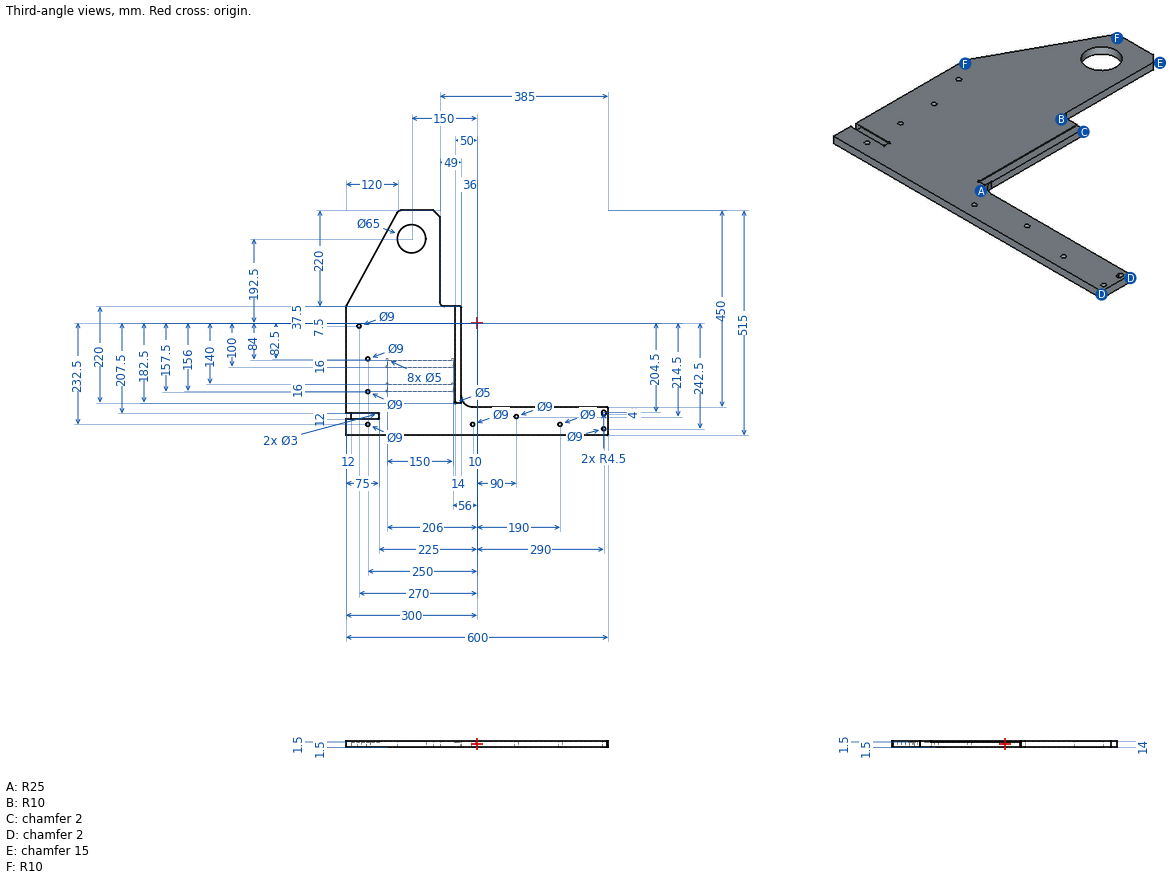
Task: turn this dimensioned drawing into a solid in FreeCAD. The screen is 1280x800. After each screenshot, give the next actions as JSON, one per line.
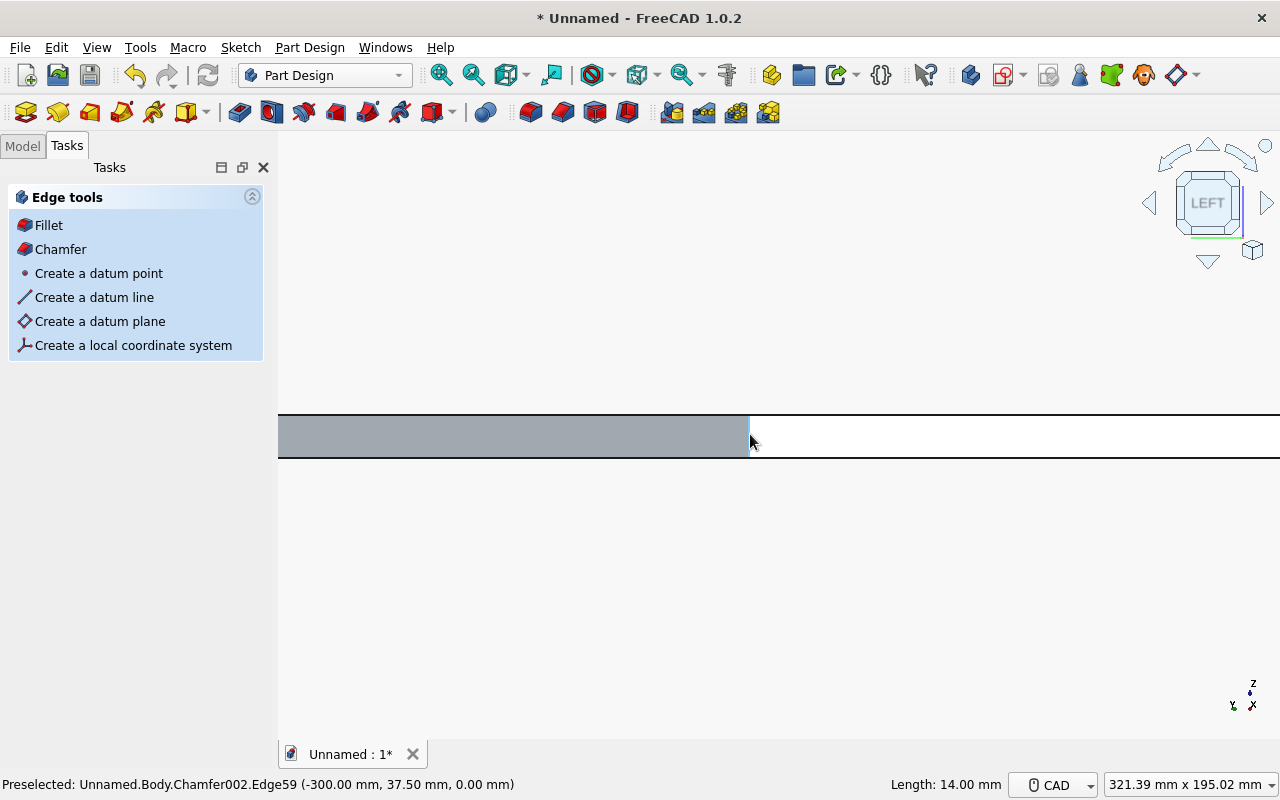
{"action": "left_click", "coordinate": [749, 436], "text": "ctrl"}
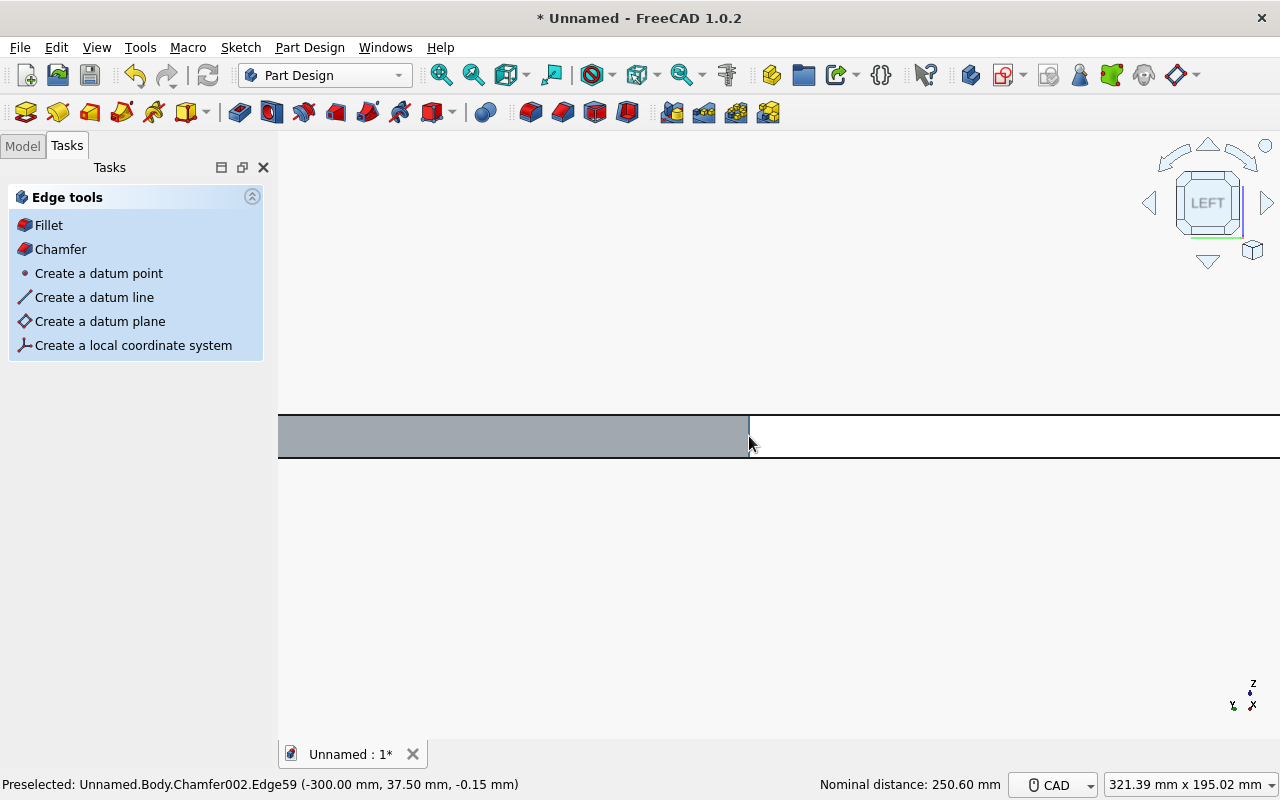
{"action": "left_click", "coordinate": [532, 112]}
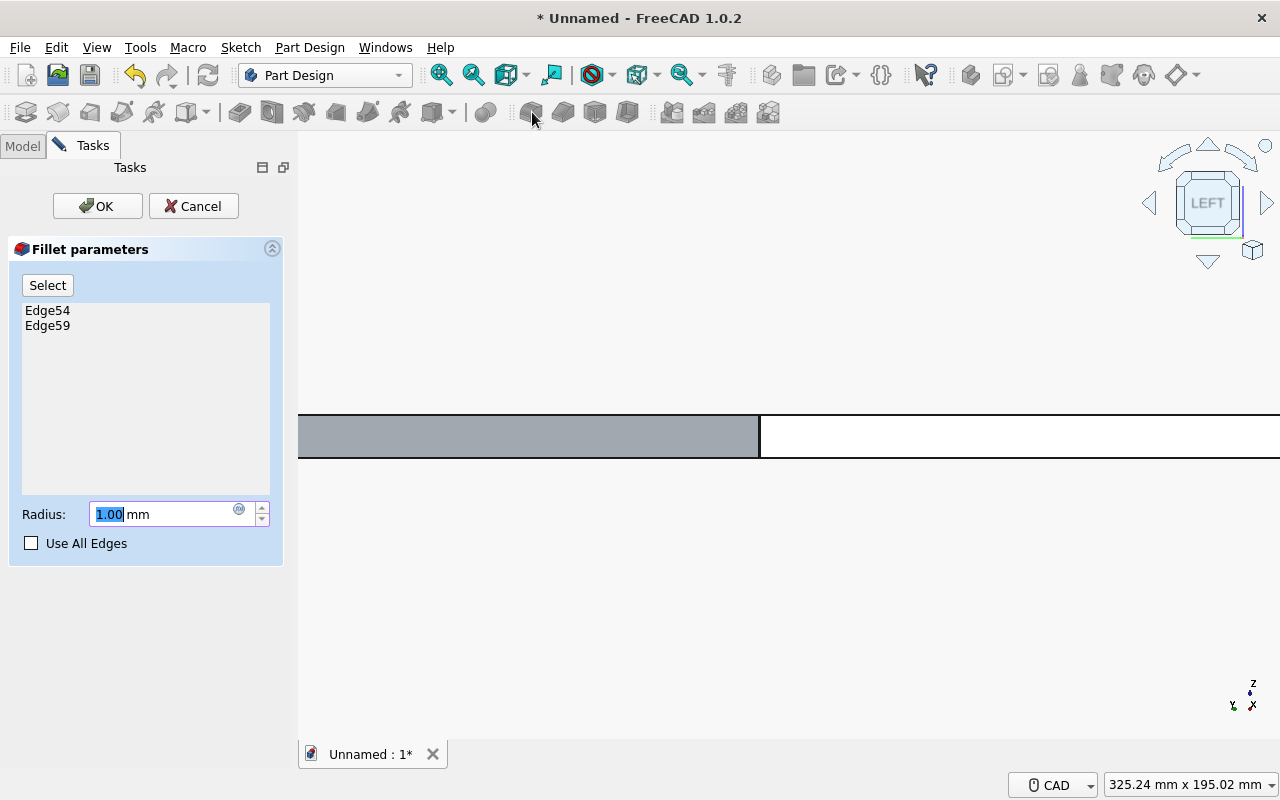
{"action": "type", "text": "10"}
{"action": "key", "text": "Tab"}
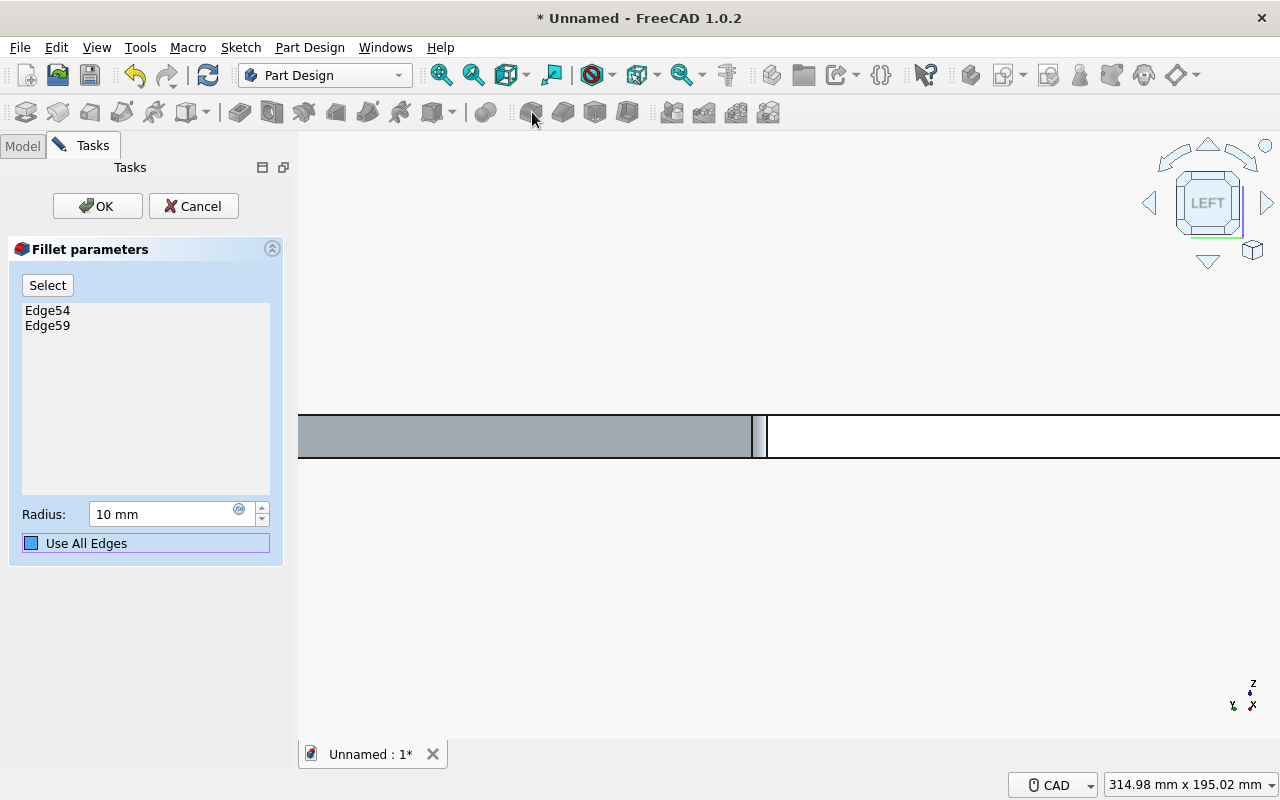
{"action": "left_click", "coordinate": [98, 206]}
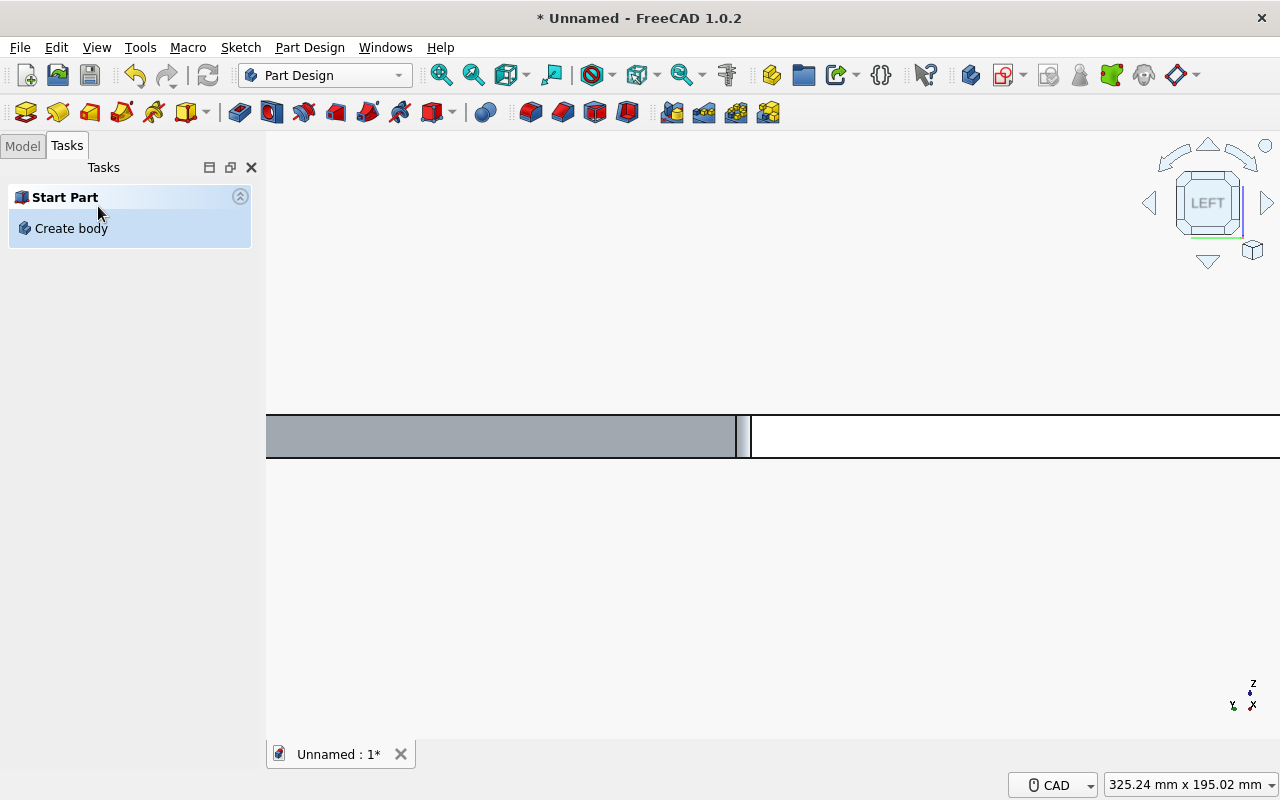
{"action": "key", "text": "0"}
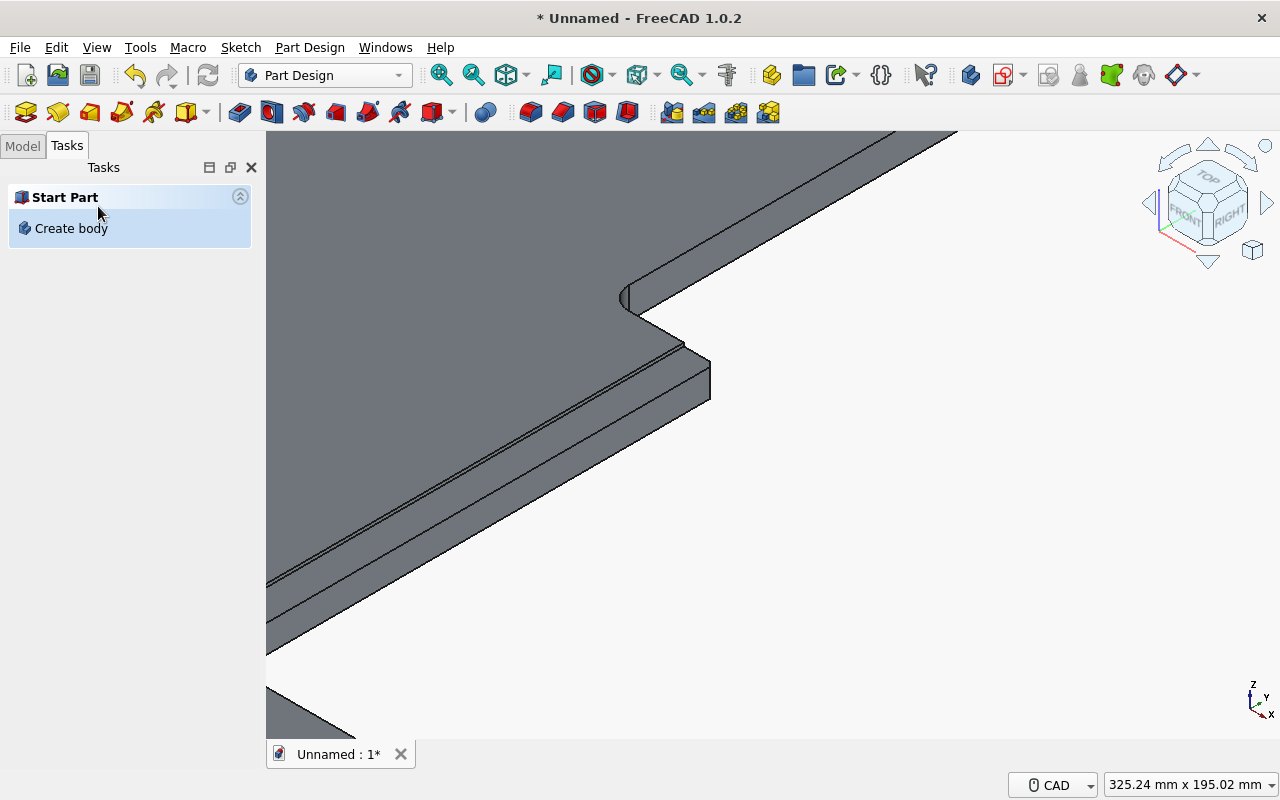
{"action": "left_click", "coordinate": [442, 76]}